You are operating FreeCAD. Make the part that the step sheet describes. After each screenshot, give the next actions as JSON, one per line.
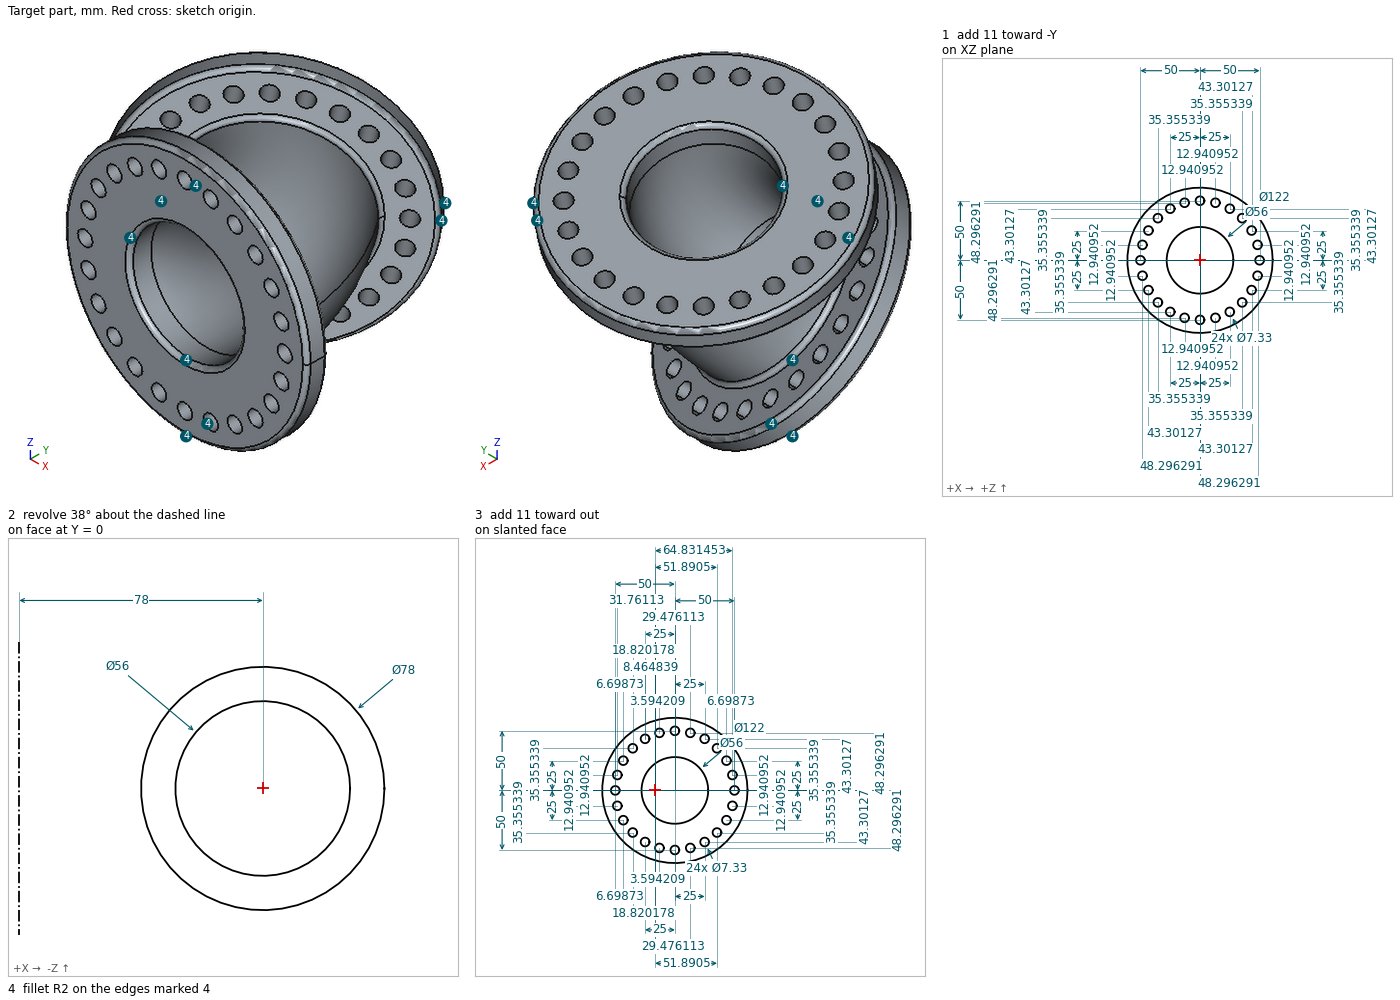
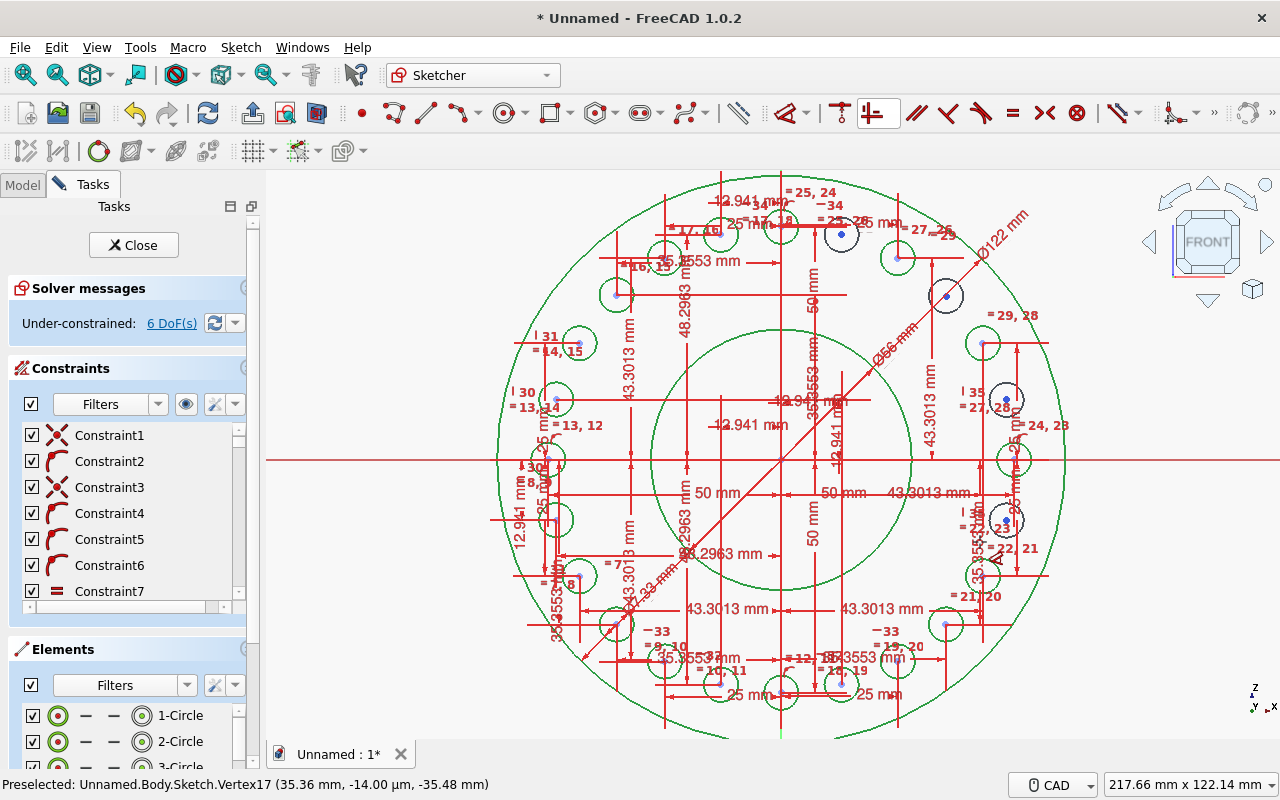
{"action": "left_click", "coordinate": [1007, 520]}
{"action": "left_click", "coordinate": [894, 554]}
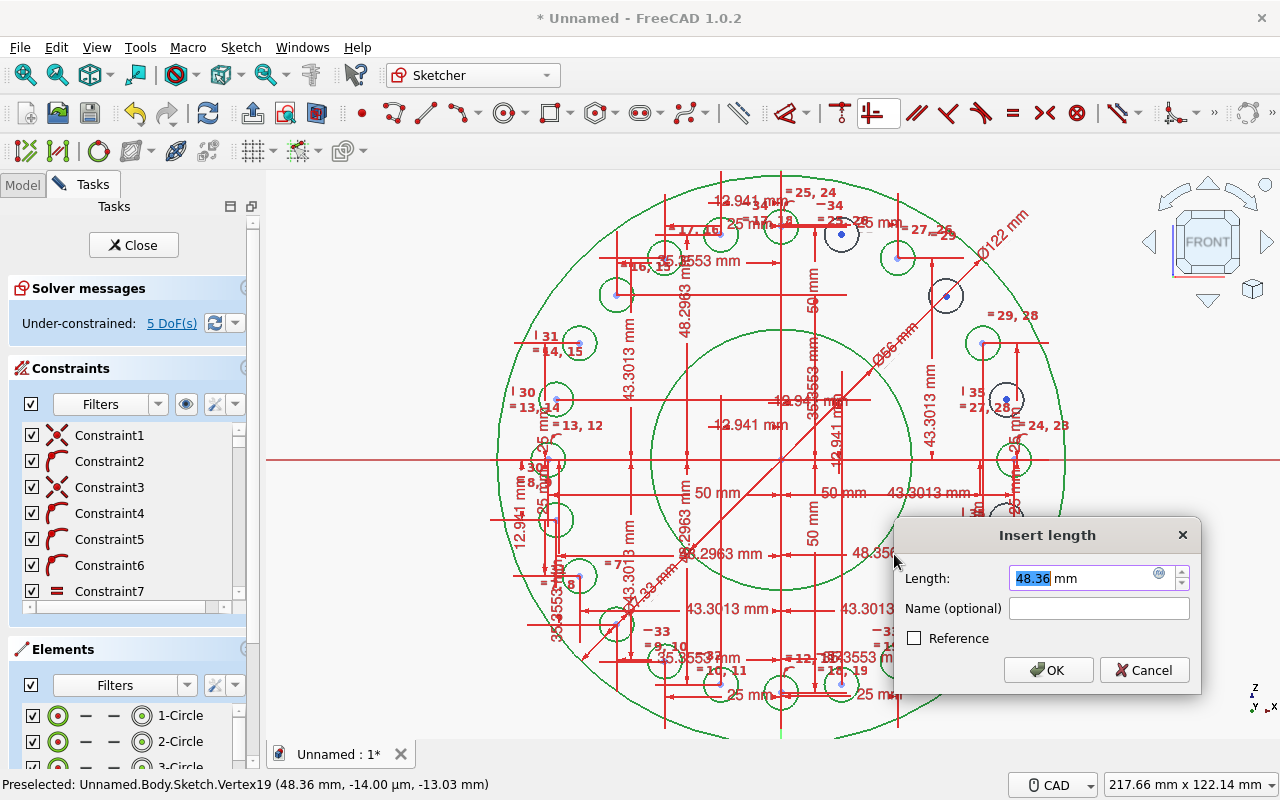
{"action": "type", "text": "48.296291"}
{"action": "key", "text": "Return"}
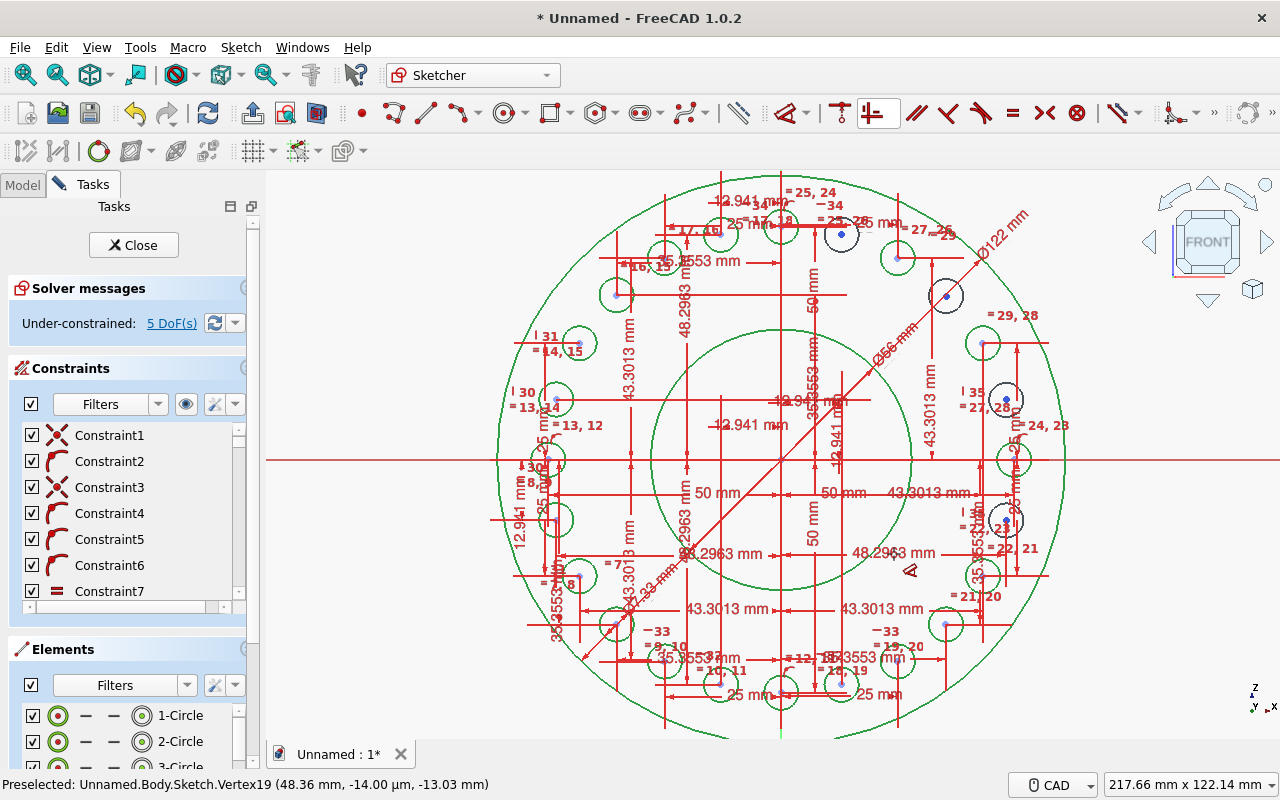
{"action": "left_click", "coordinate": [1006, 520]}
{"action": "left_click", "coordinate": [1040, 511]}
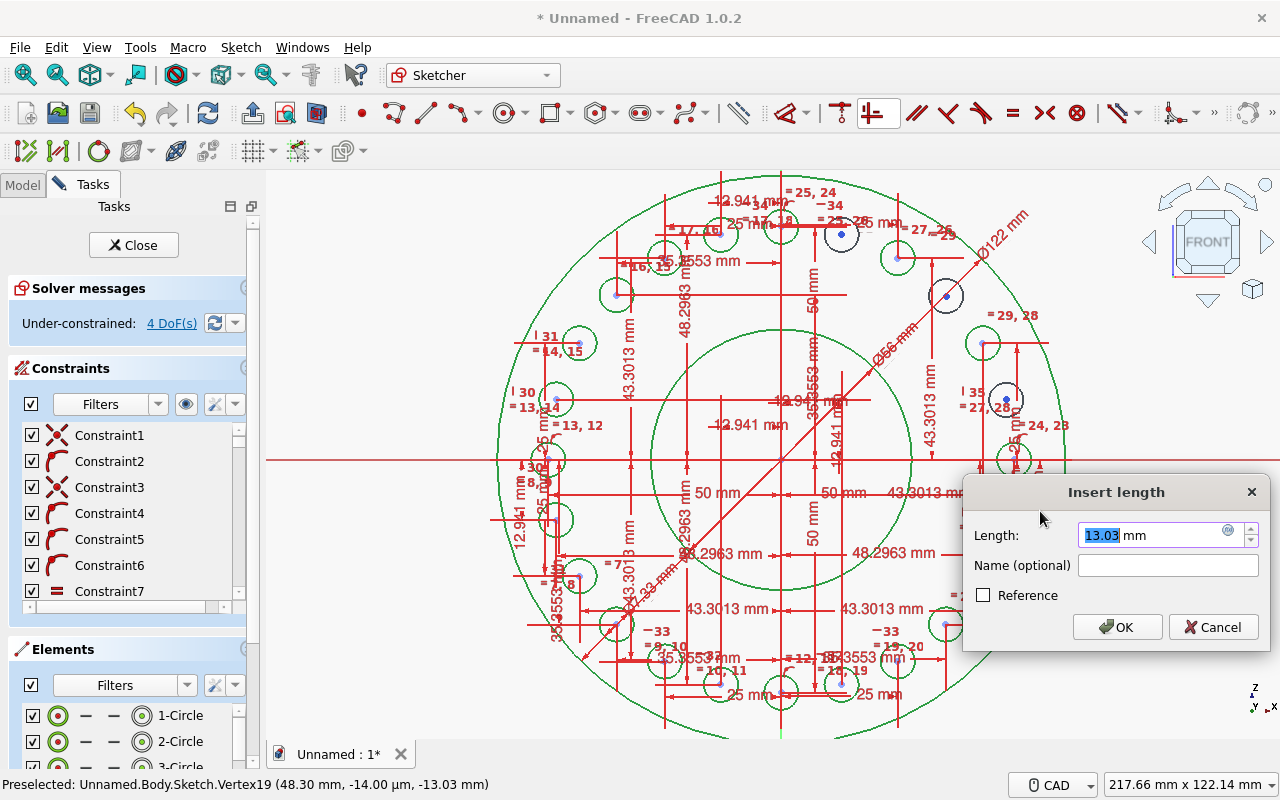
{"action": "type", "text": "12.940952"}
{"action": "key", "text": "Return"}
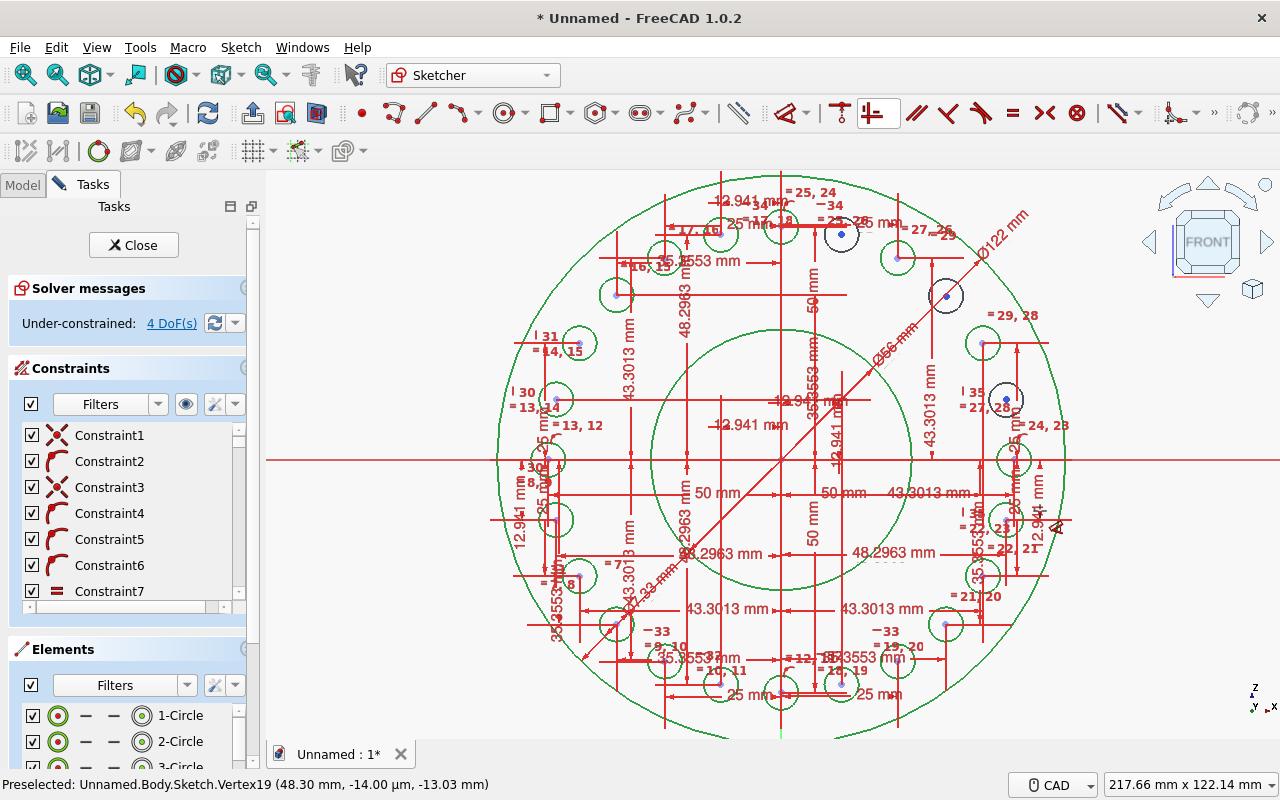
{"action": "left_click", "coordinate": [842, 235]}
{"action": "left_click", "coordinate": [825, 201]}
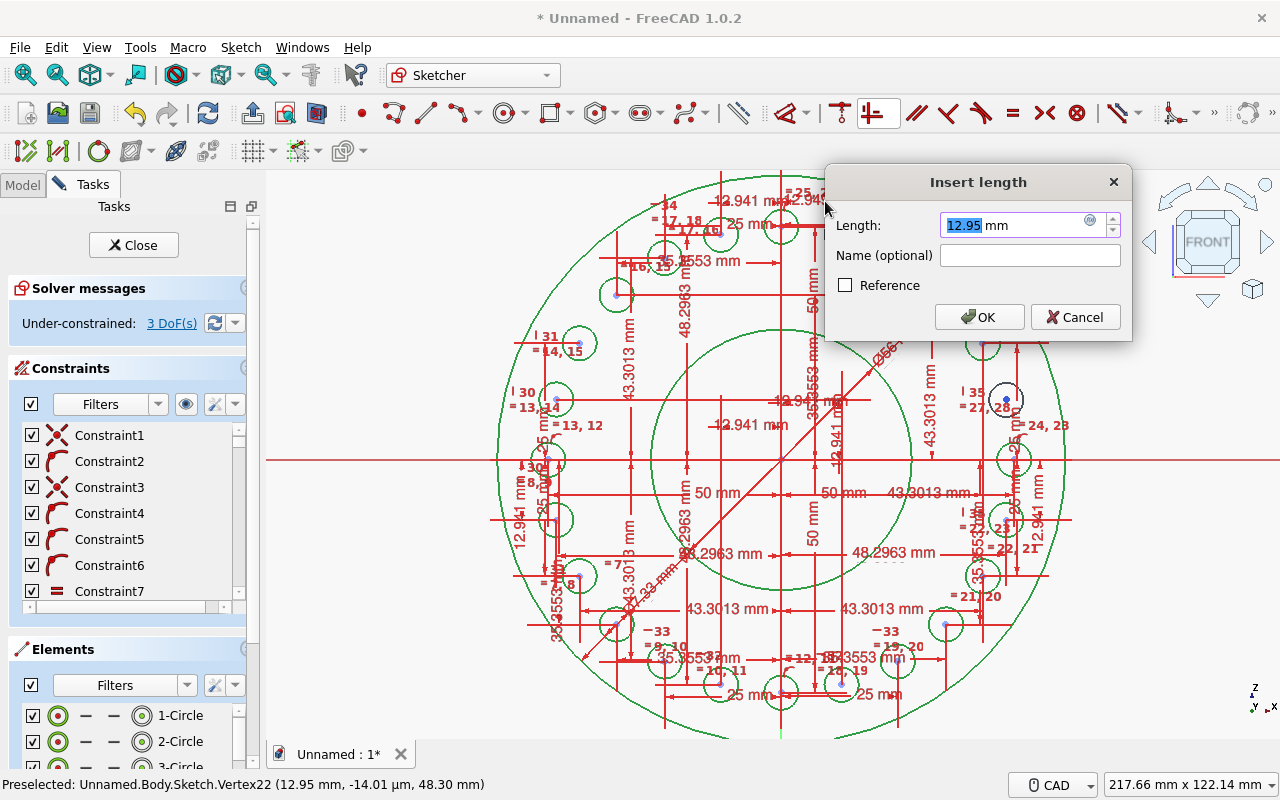
{"action": "type", "text": "12.940952"}
{"action": "key", "text": "Return"}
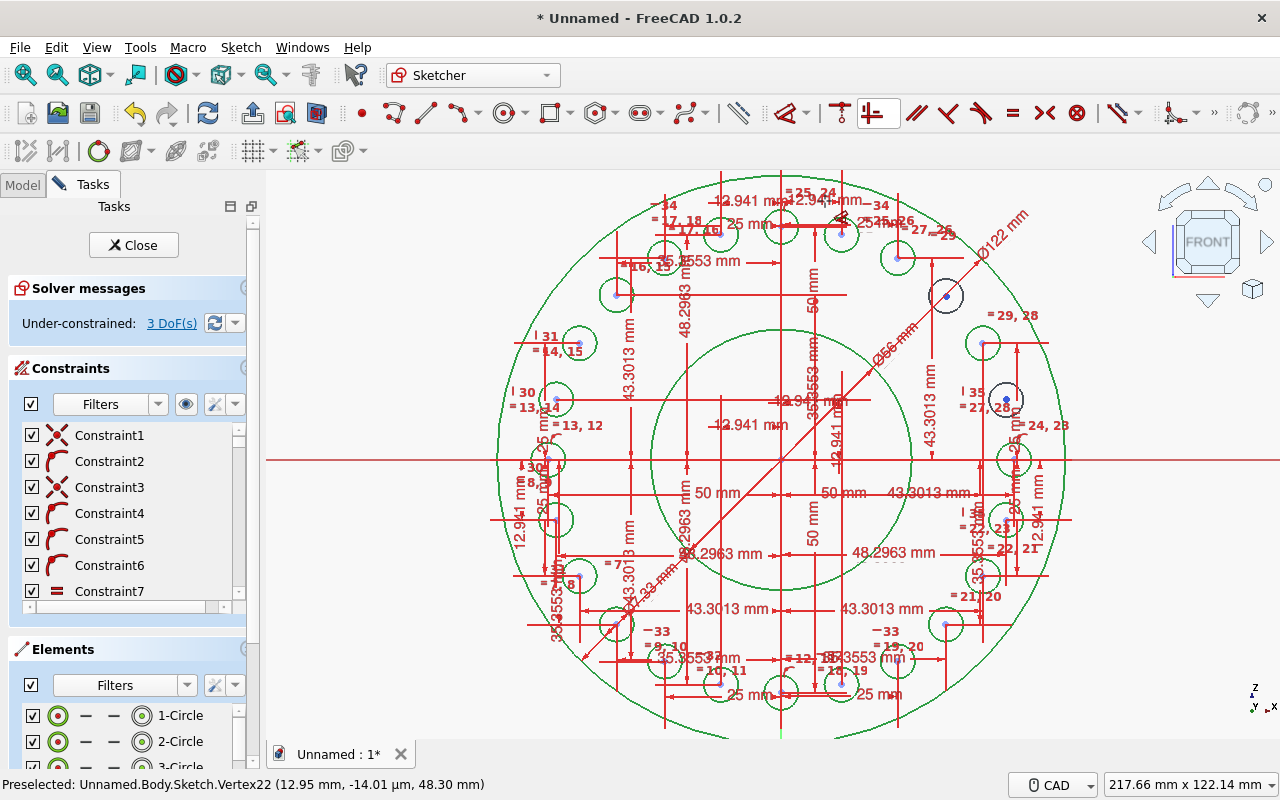
{"action": "left_click", "coordinate": [1006, 400]}
{"action": "left_click", "coordinate": [1088, 430]}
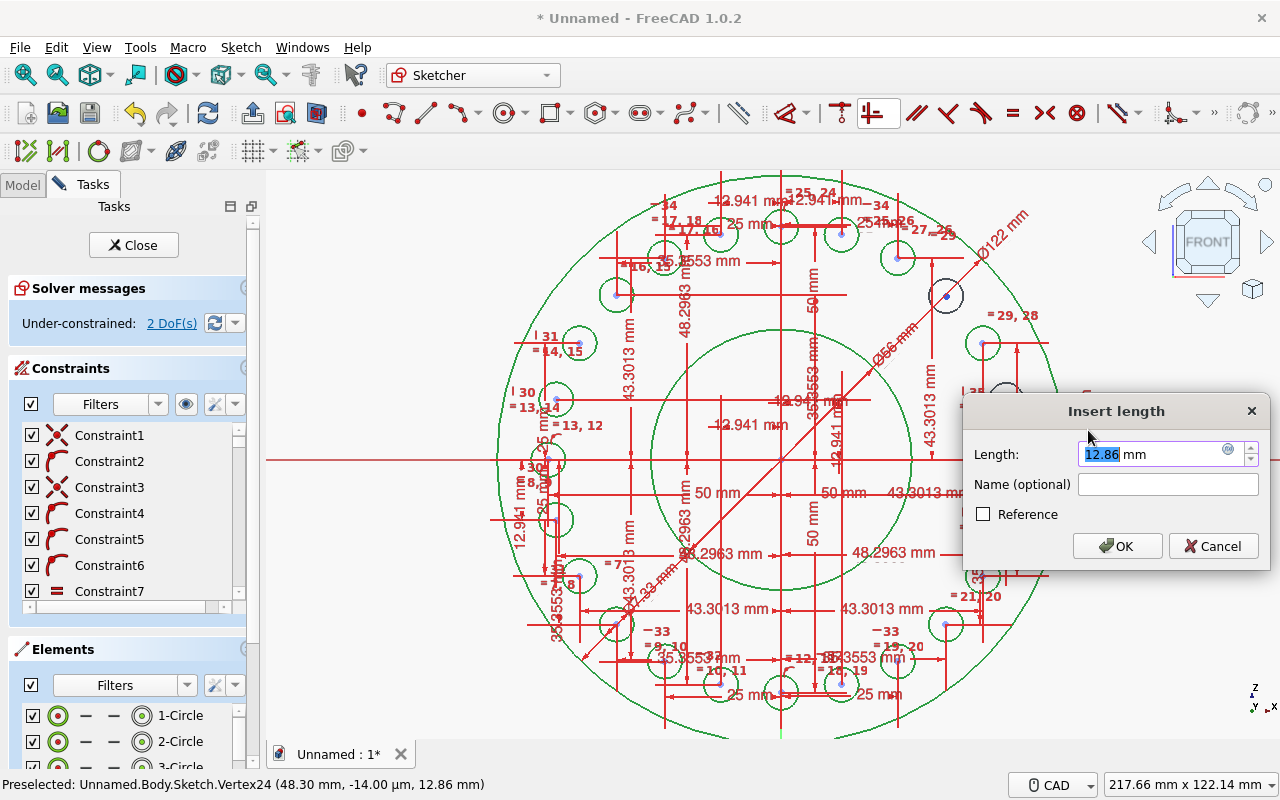
{"action": "type", "text": "12.940952"}
{"action": "key", "text": "Return"}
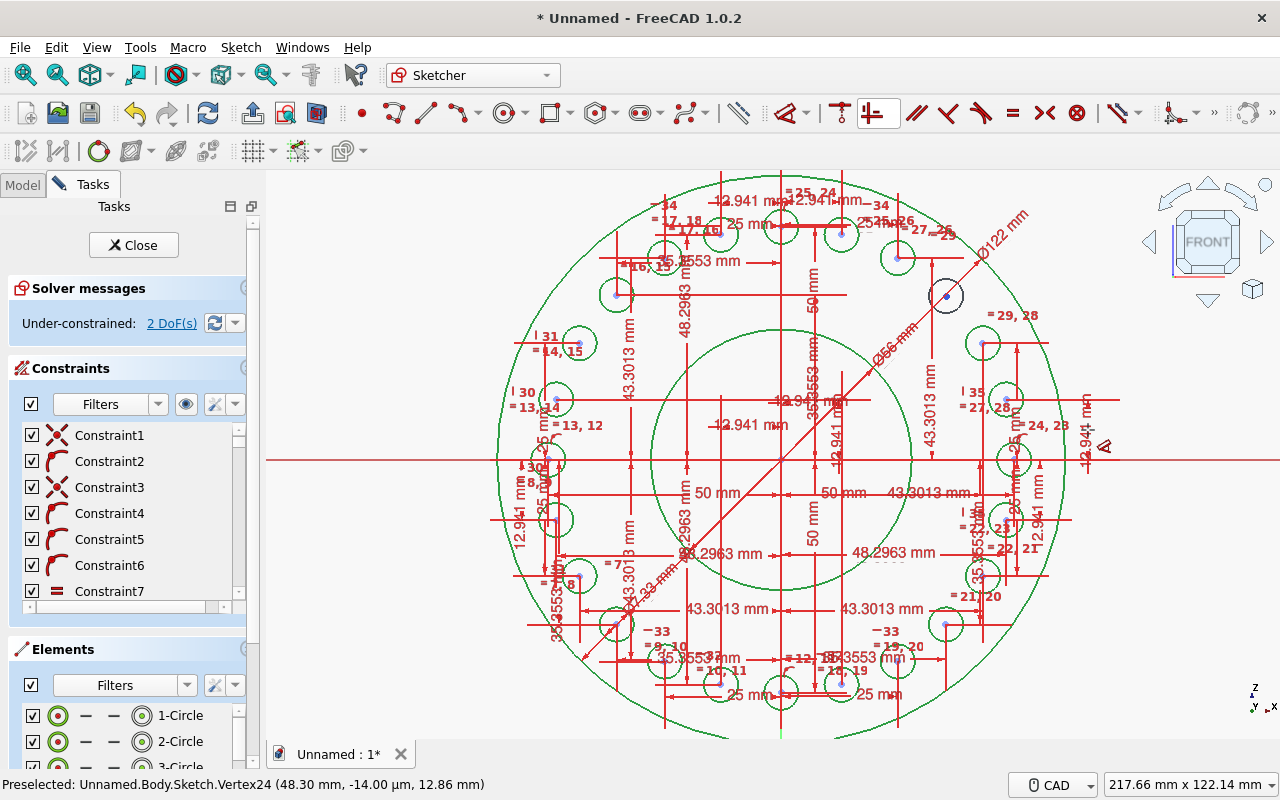
{"action": "left_click", "coordinate": [946, 296]}
{"action": "left_click", "coordinate": [864, 262]}